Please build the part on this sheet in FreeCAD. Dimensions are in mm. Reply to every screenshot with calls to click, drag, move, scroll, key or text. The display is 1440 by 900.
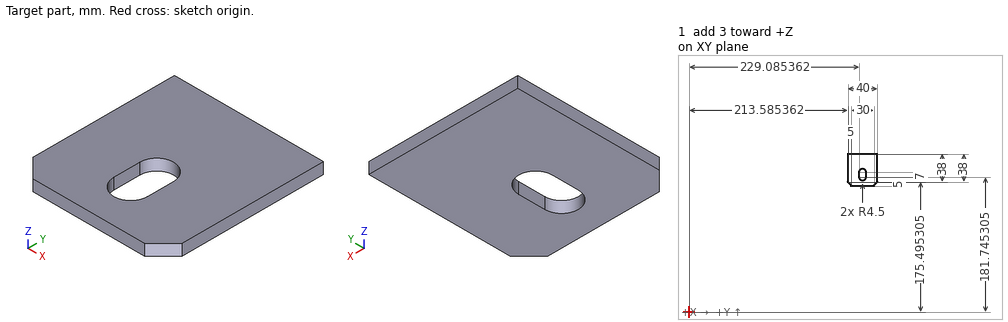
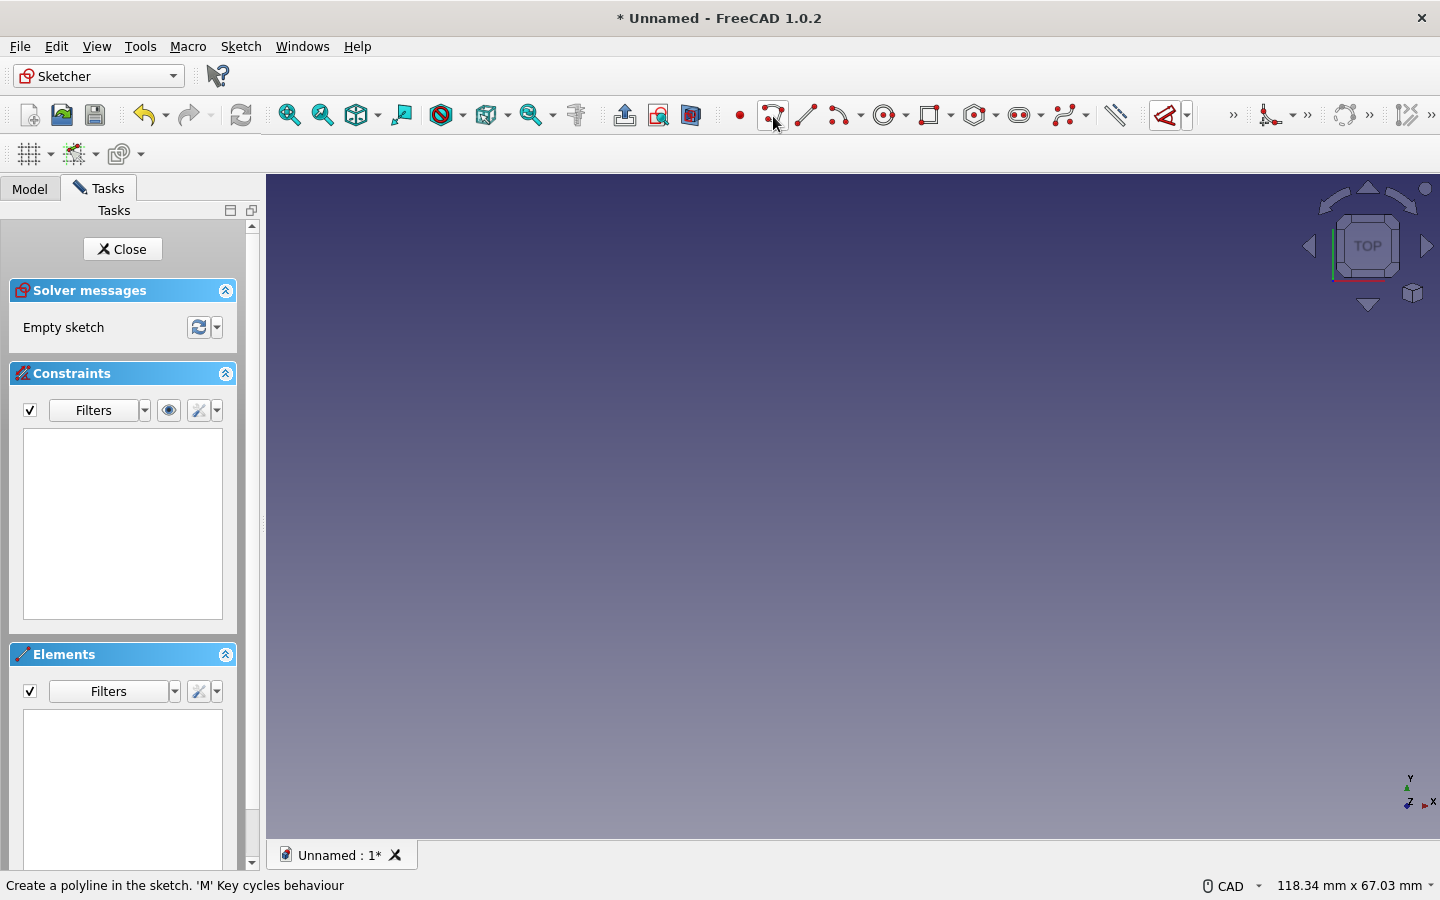
click(578, 673)
click(628, 722)
click(925, 722)
click(975, 673)
click(975, 296)
click(578, 296)
click(578, 674)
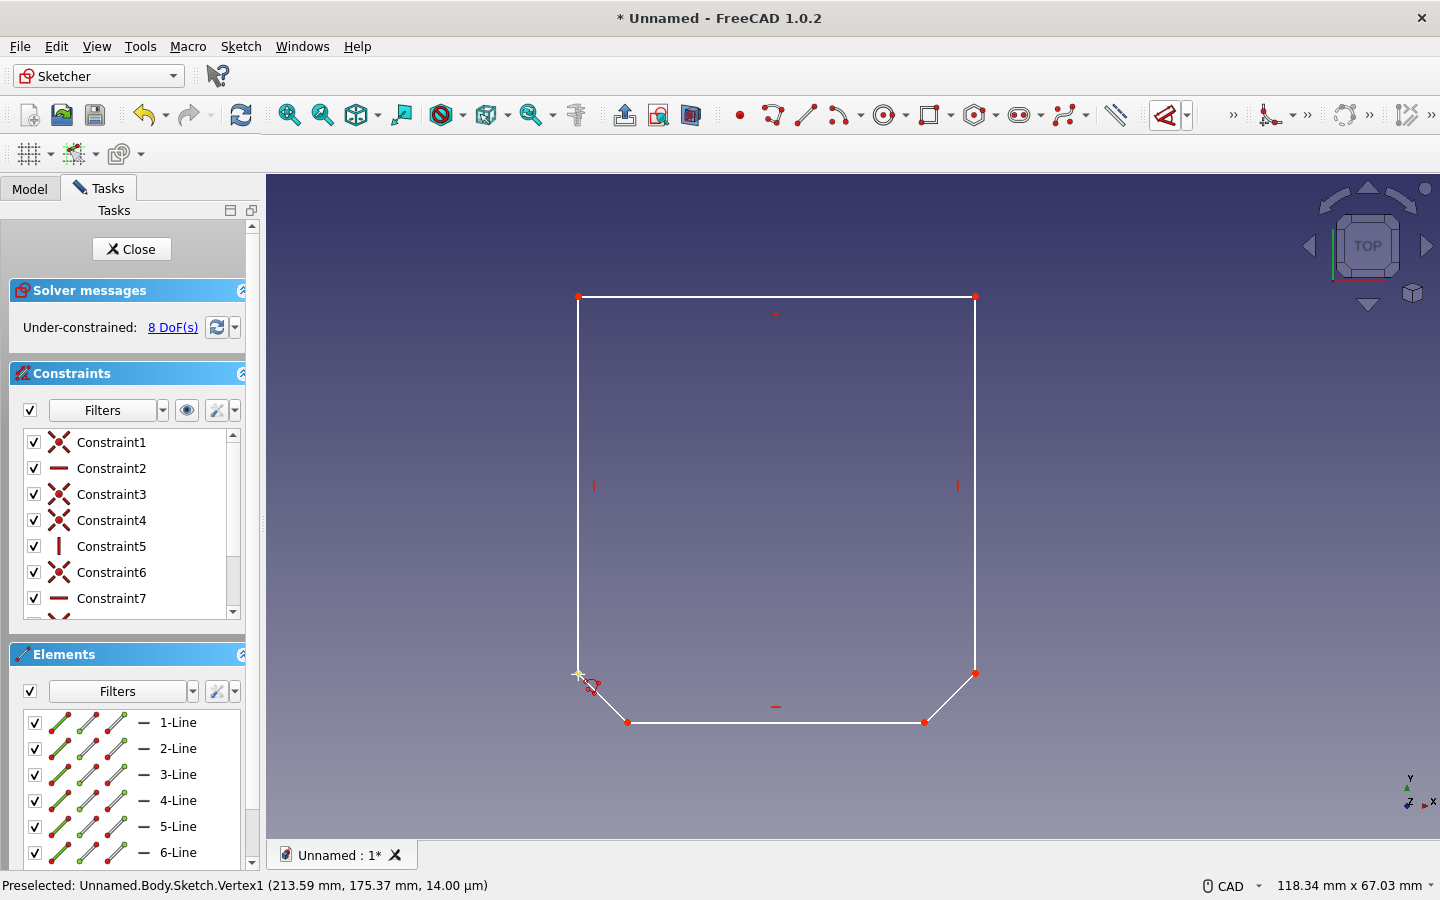
click(1018, 116)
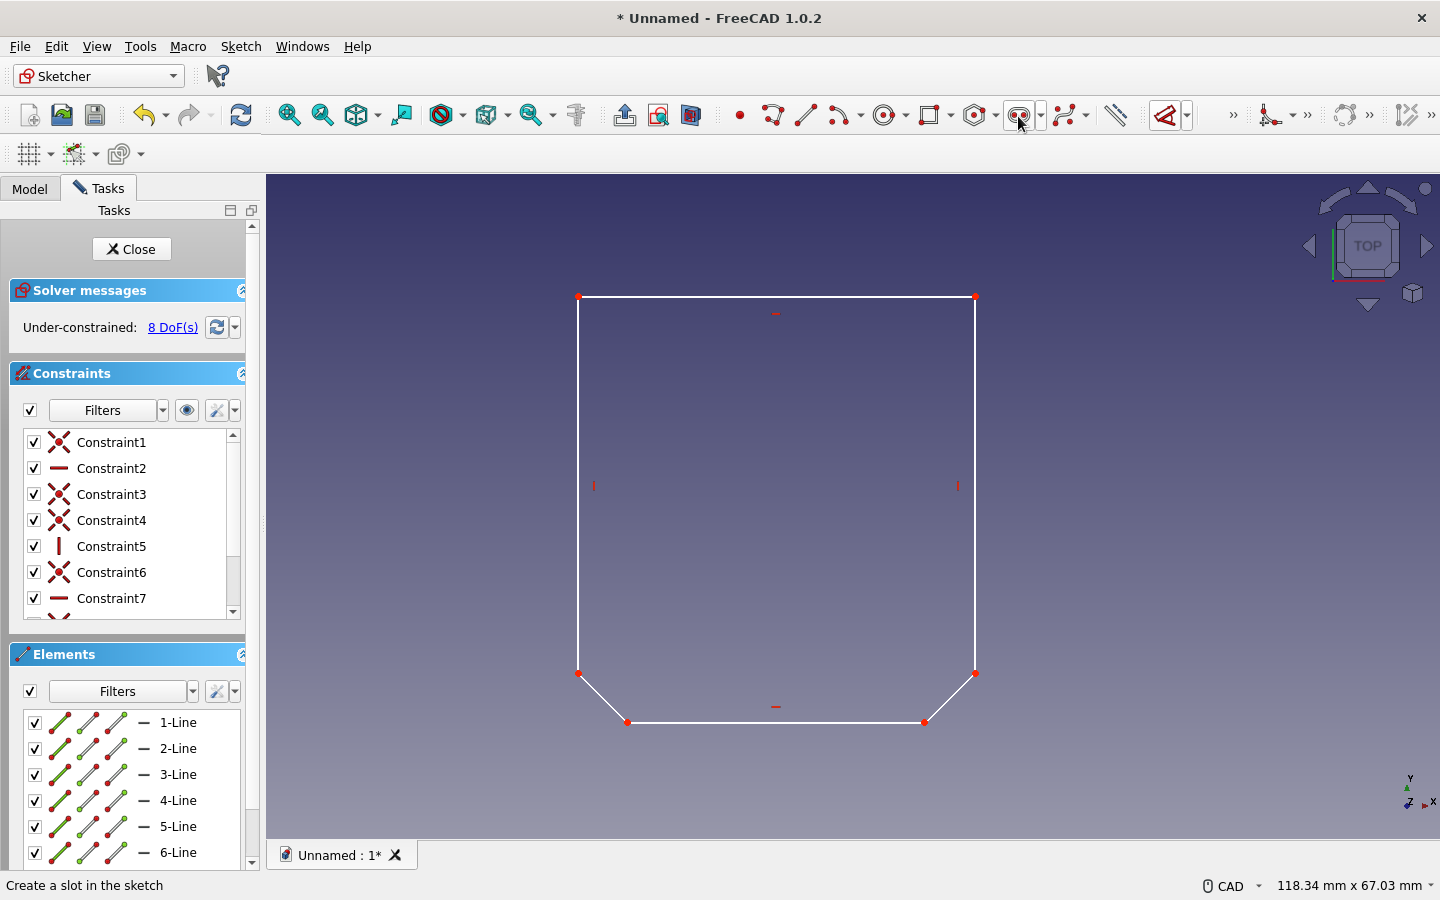
click(776, 611)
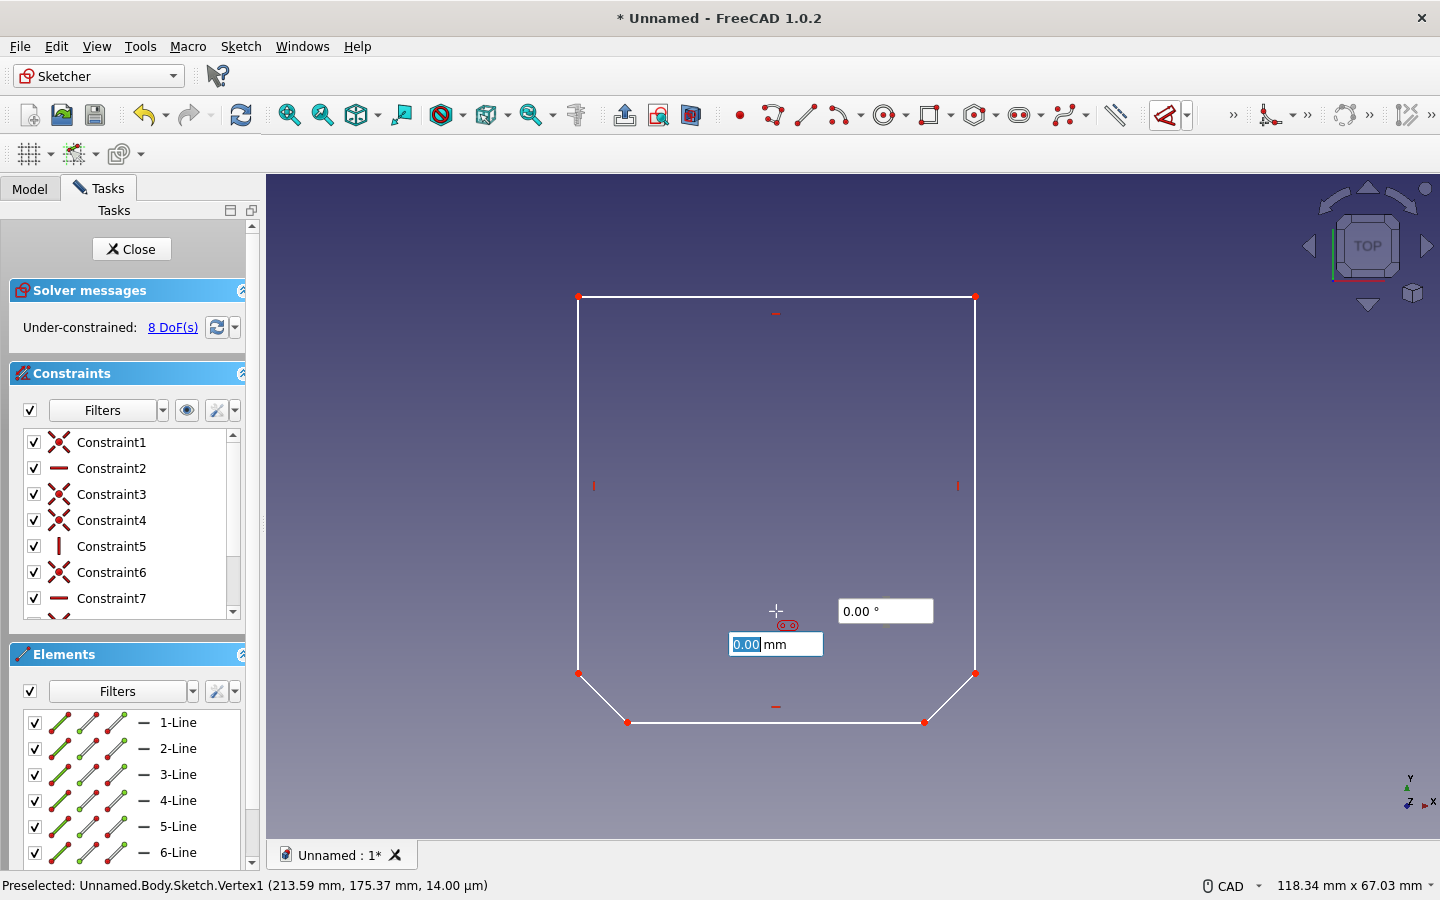
click(776, 541)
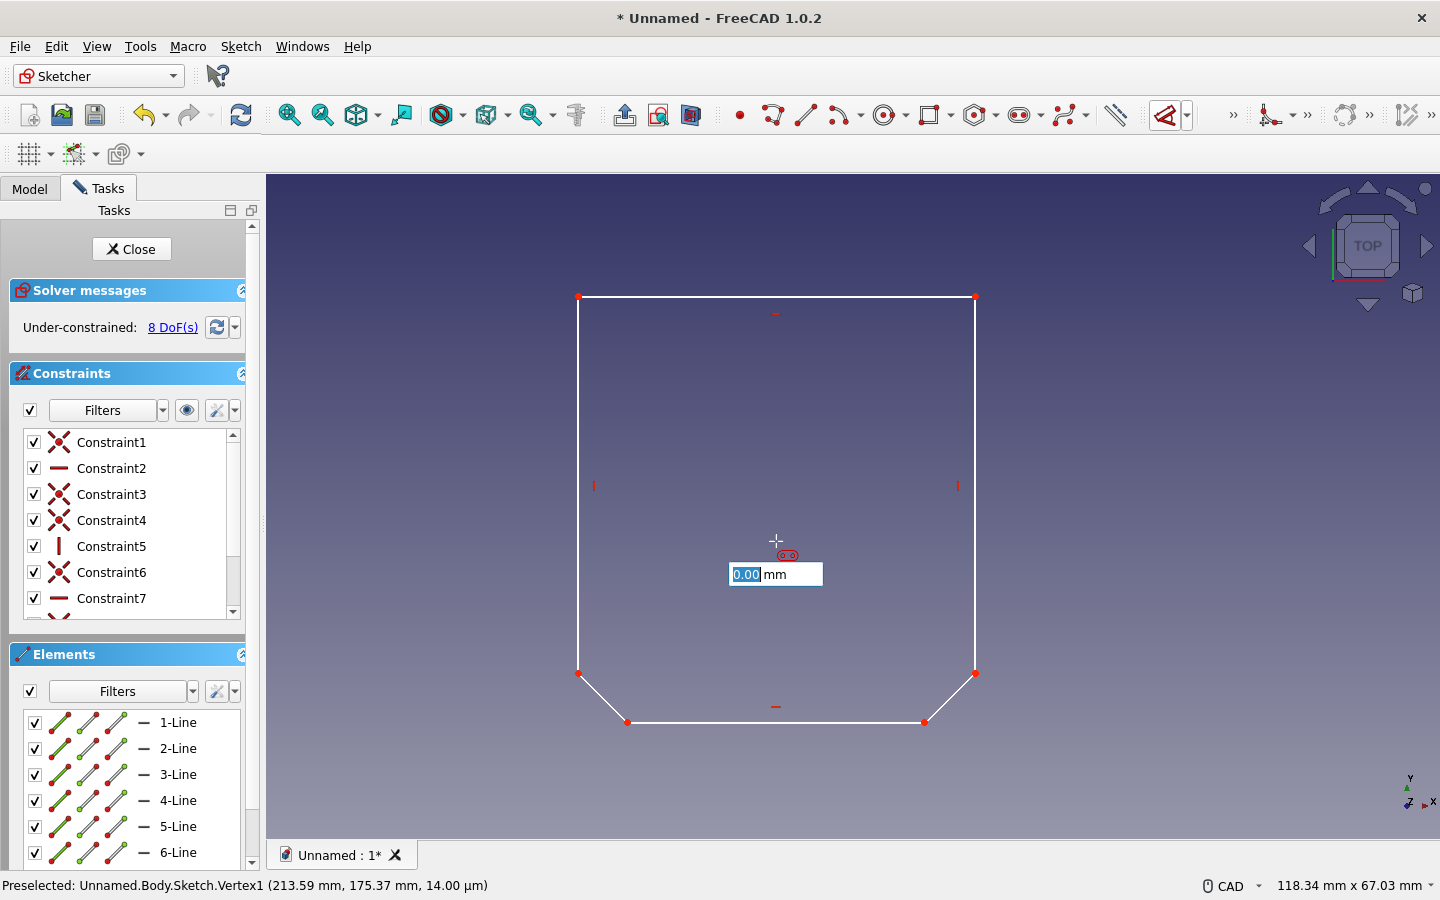
click(732, 576)
key(Escape)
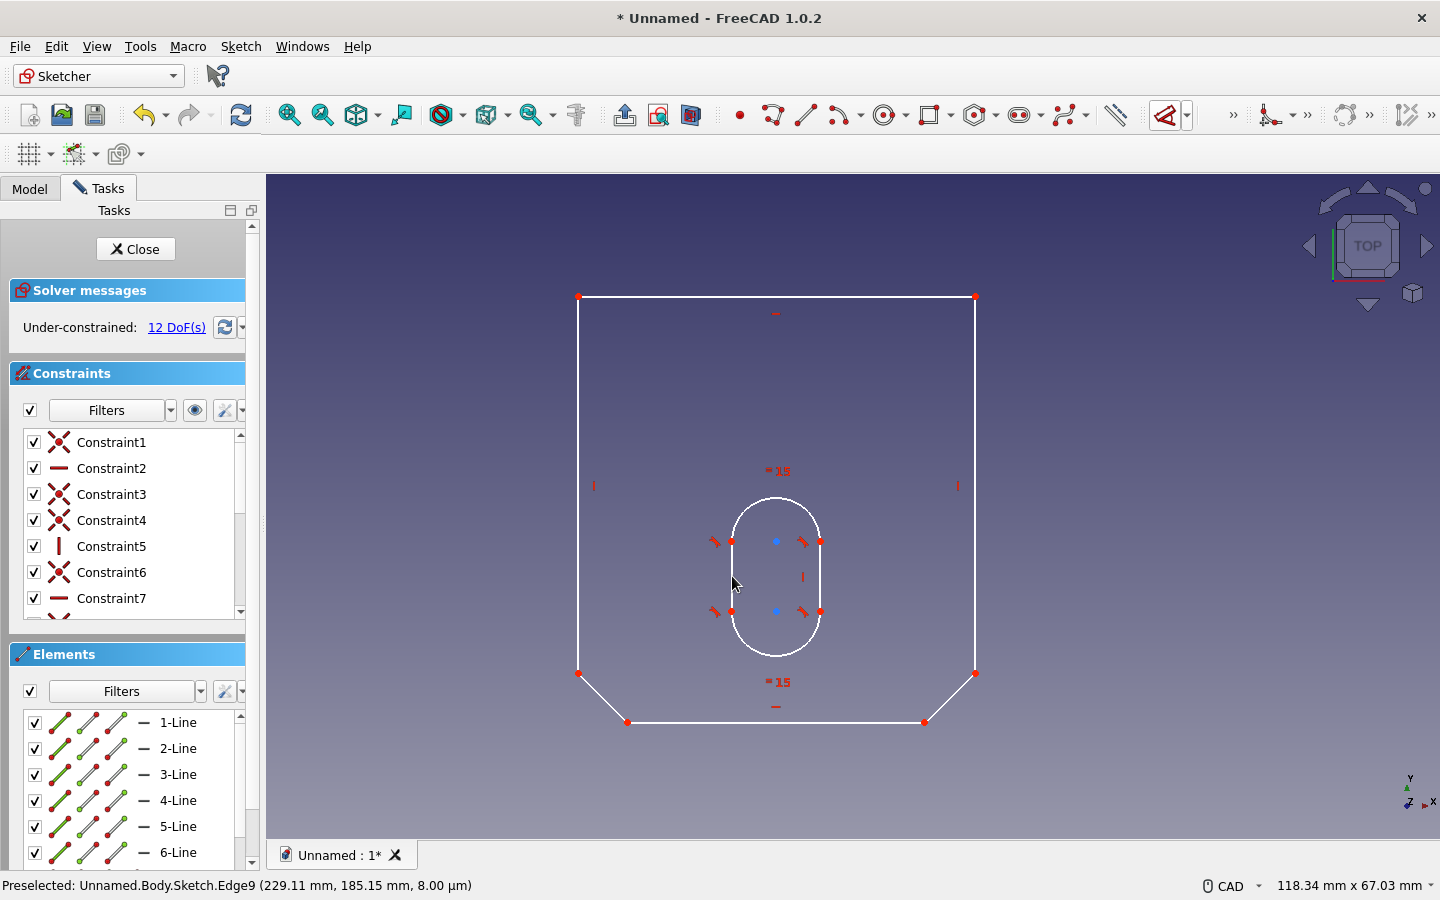
click(1164, 116)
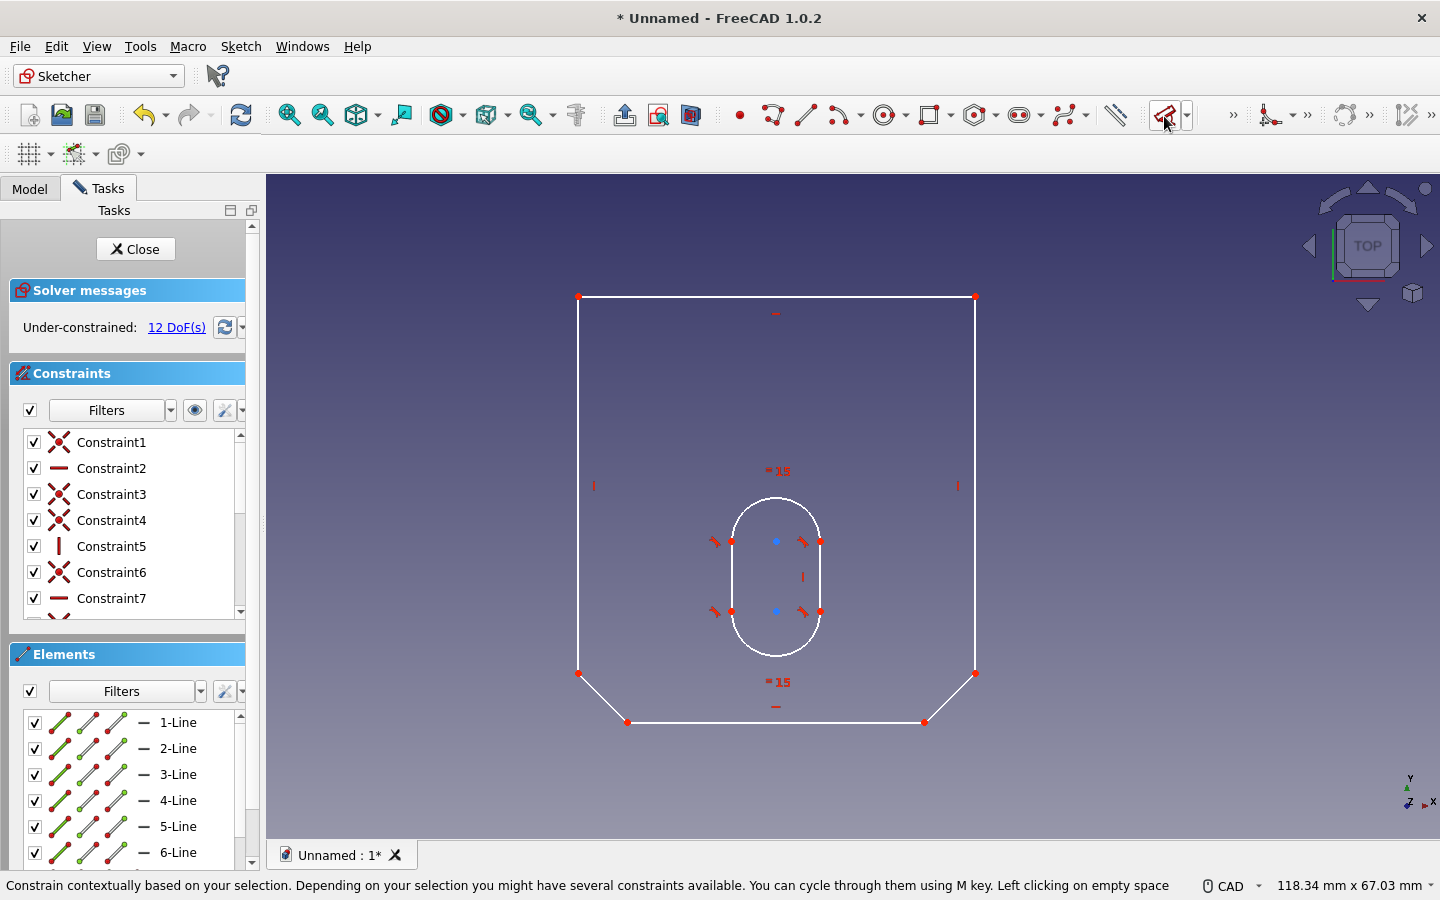
click(750, 648)
click(731, 674)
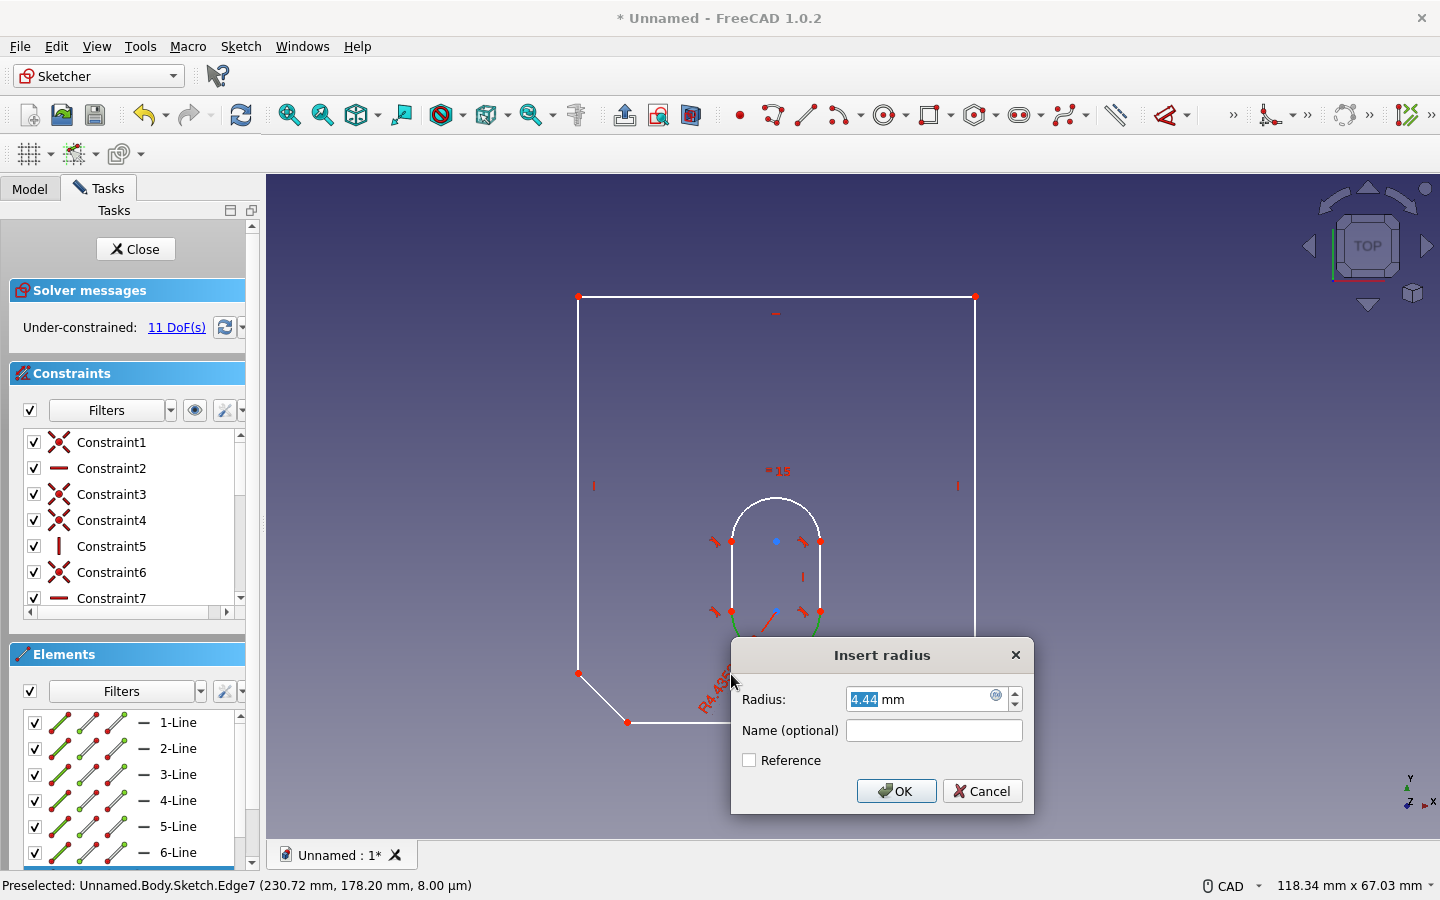
text(4.5)
key(Return)